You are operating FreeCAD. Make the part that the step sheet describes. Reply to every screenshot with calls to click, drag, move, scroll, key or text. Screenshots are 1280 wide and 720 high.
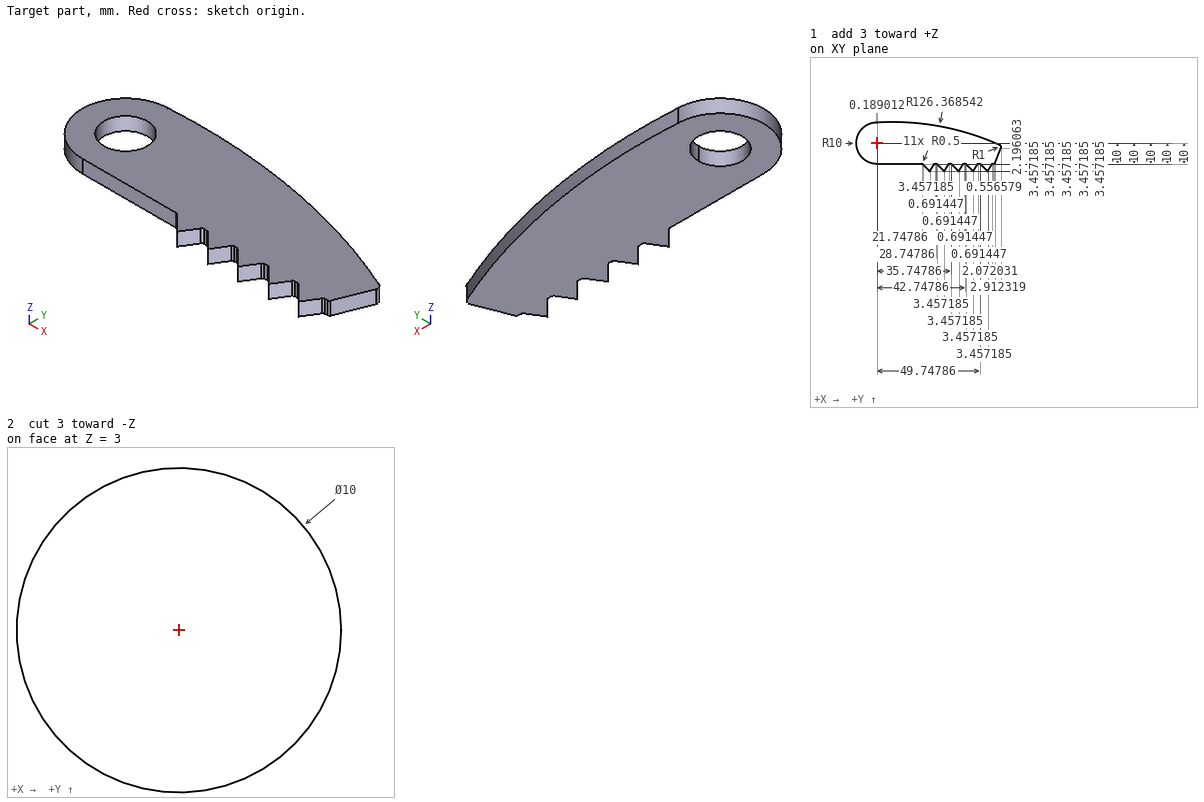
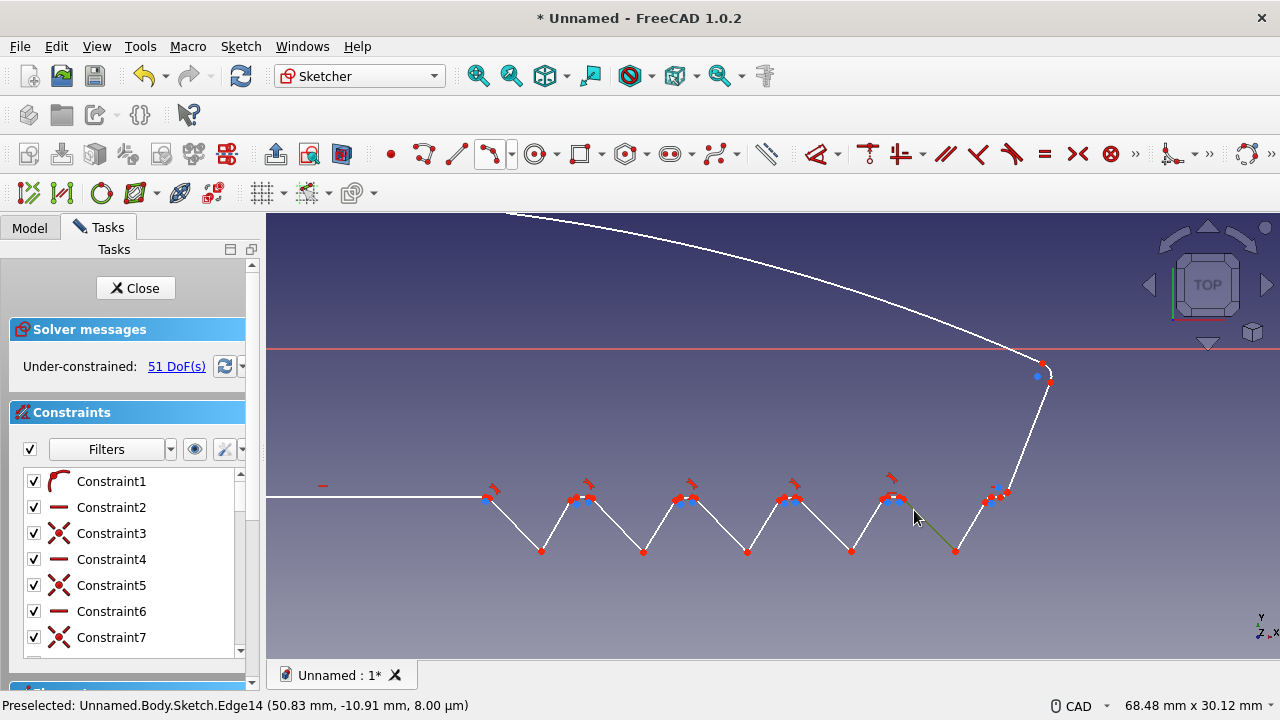
scroll(902, 498, up, 9)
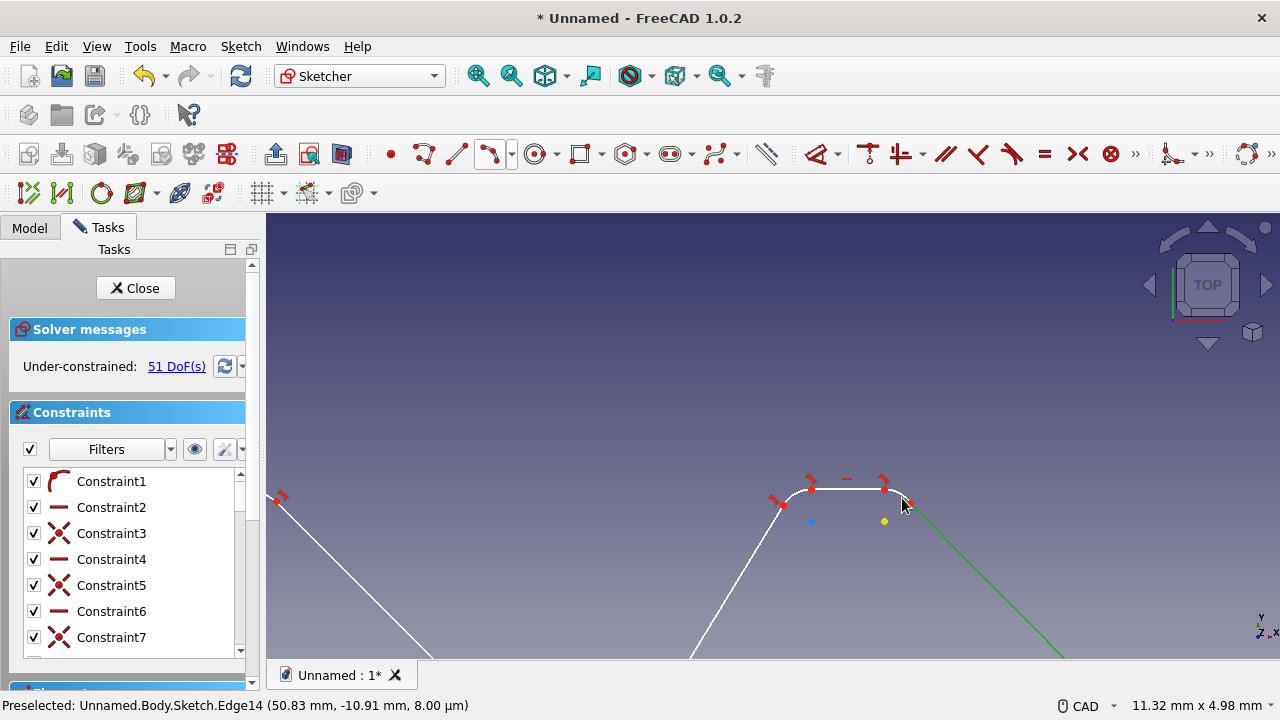
click(899, 493)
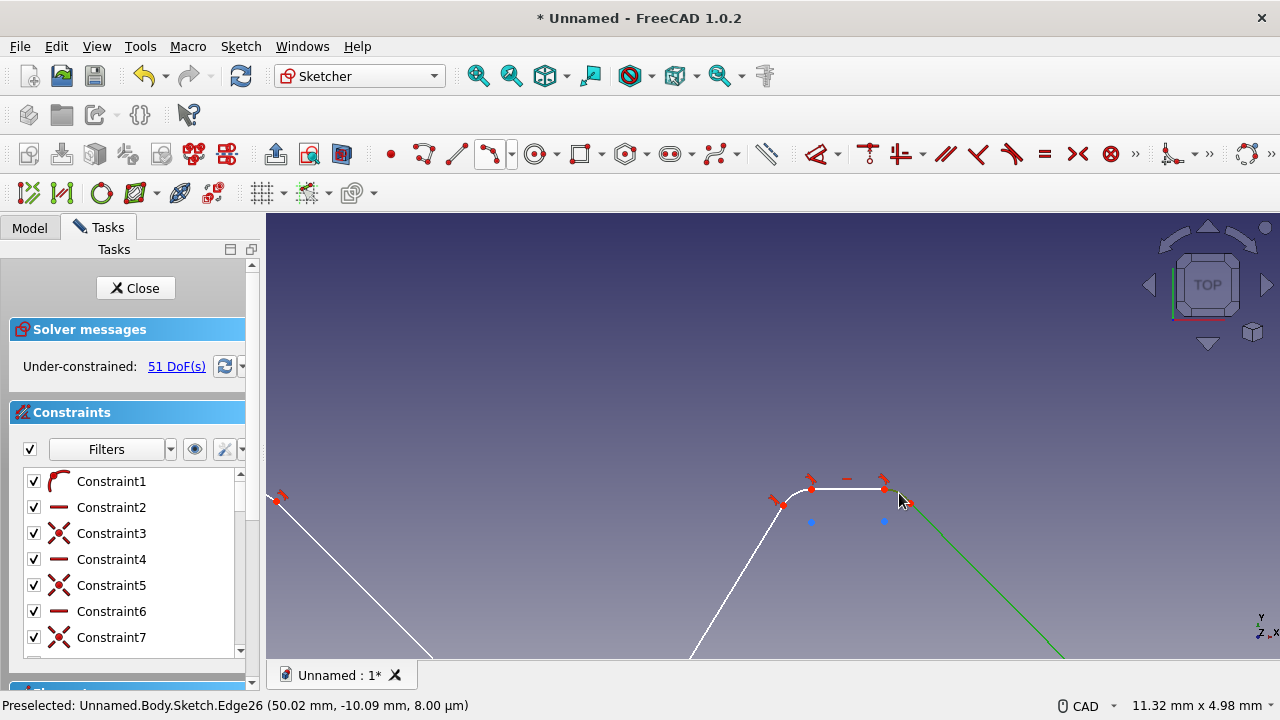
click(1012, 154)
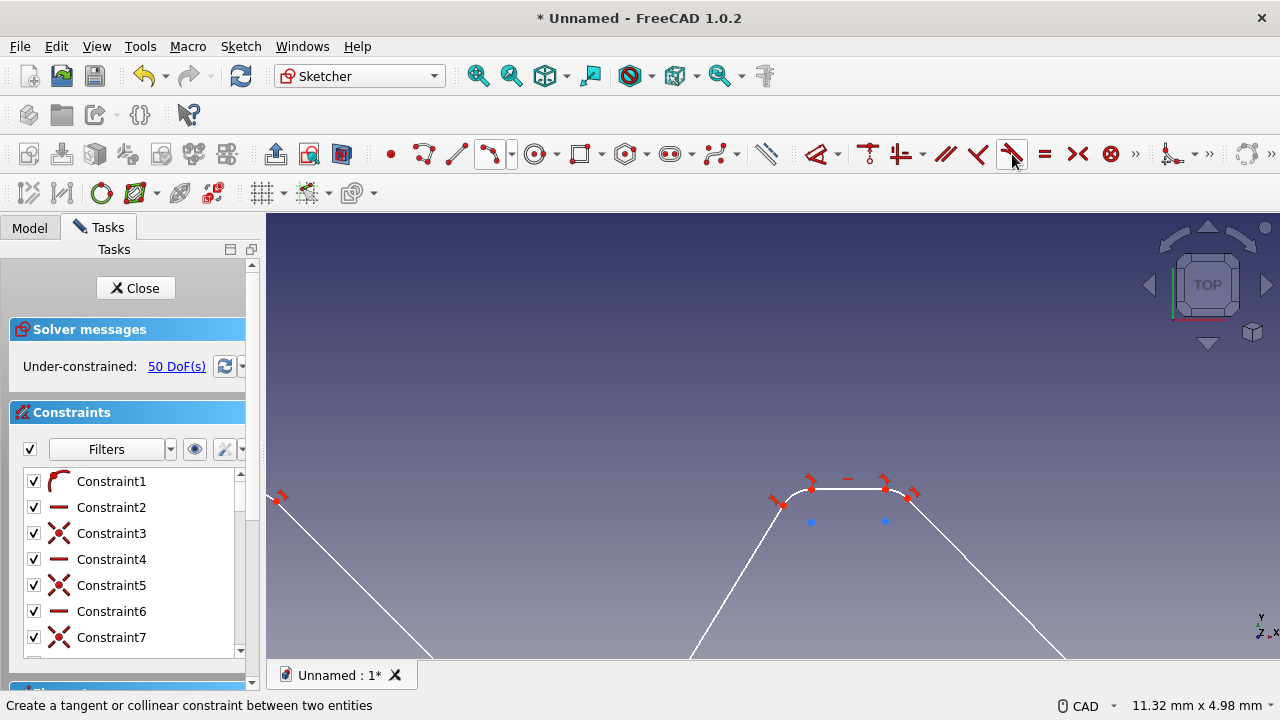
scroll(908, 504, down, 12)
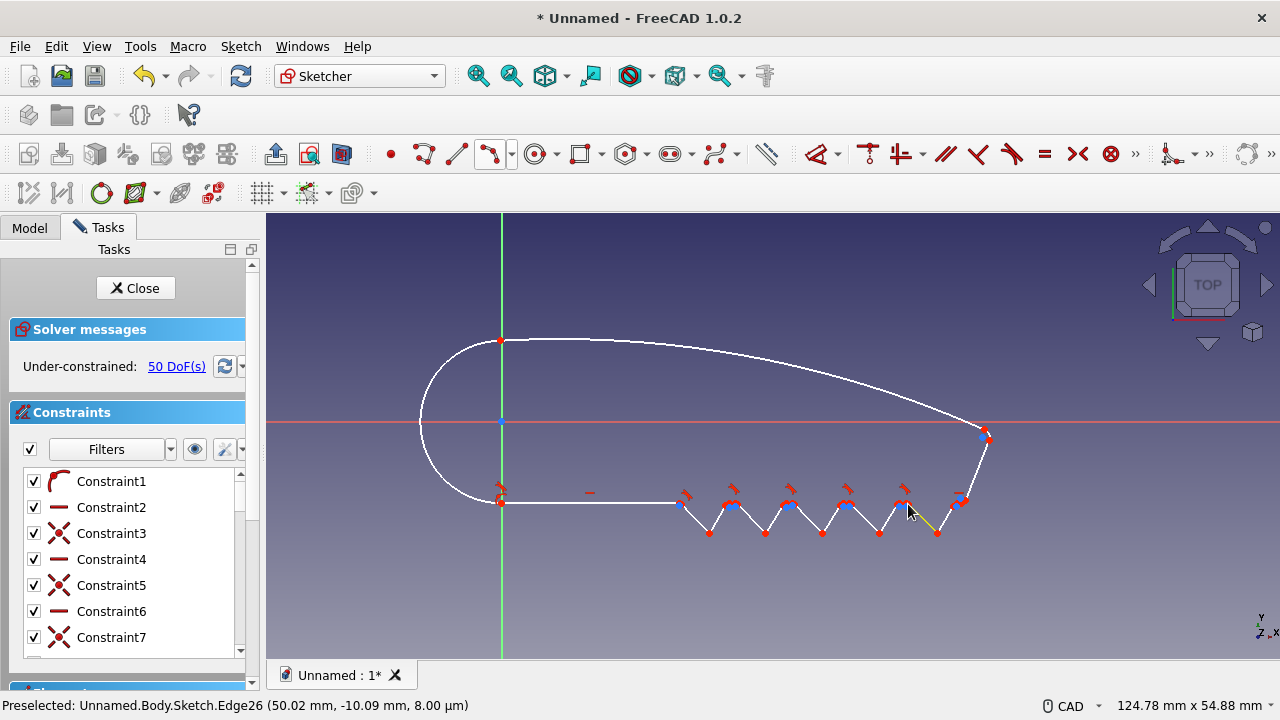
scroll(942, 525, up, 3)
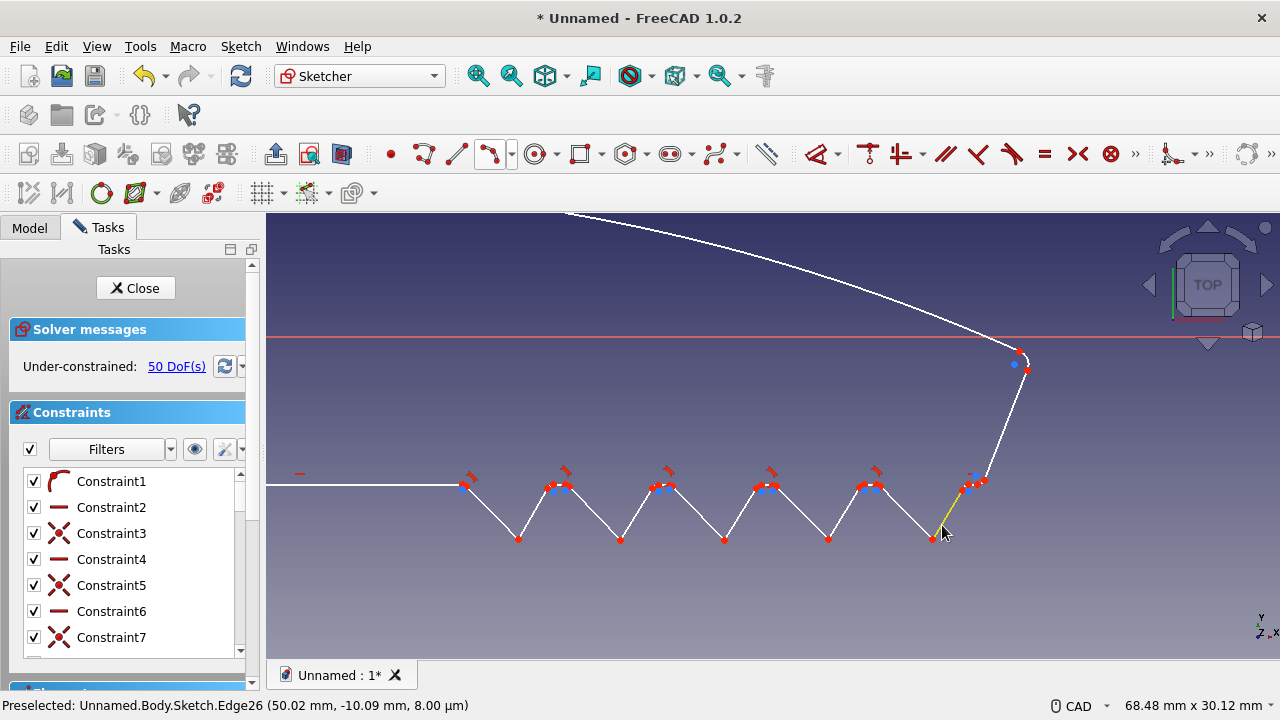
click(942, 525)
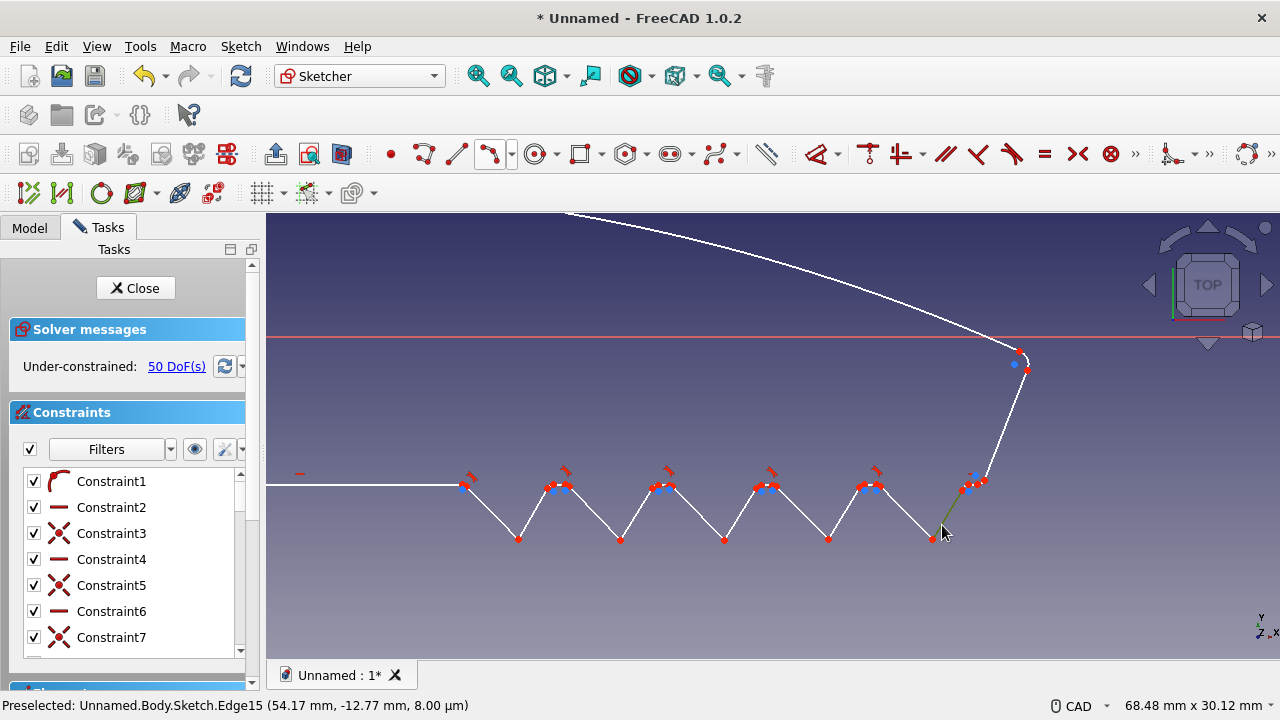
scroll(964, 486, up, 6)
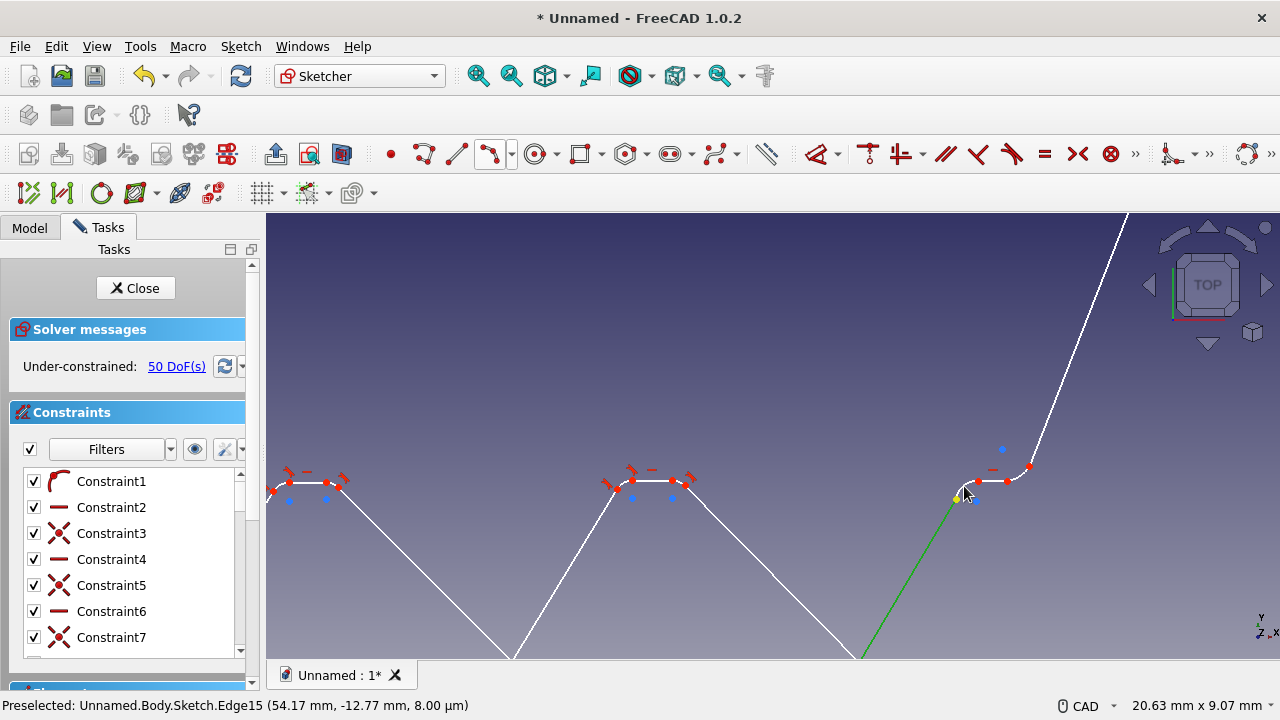
click(964, 485)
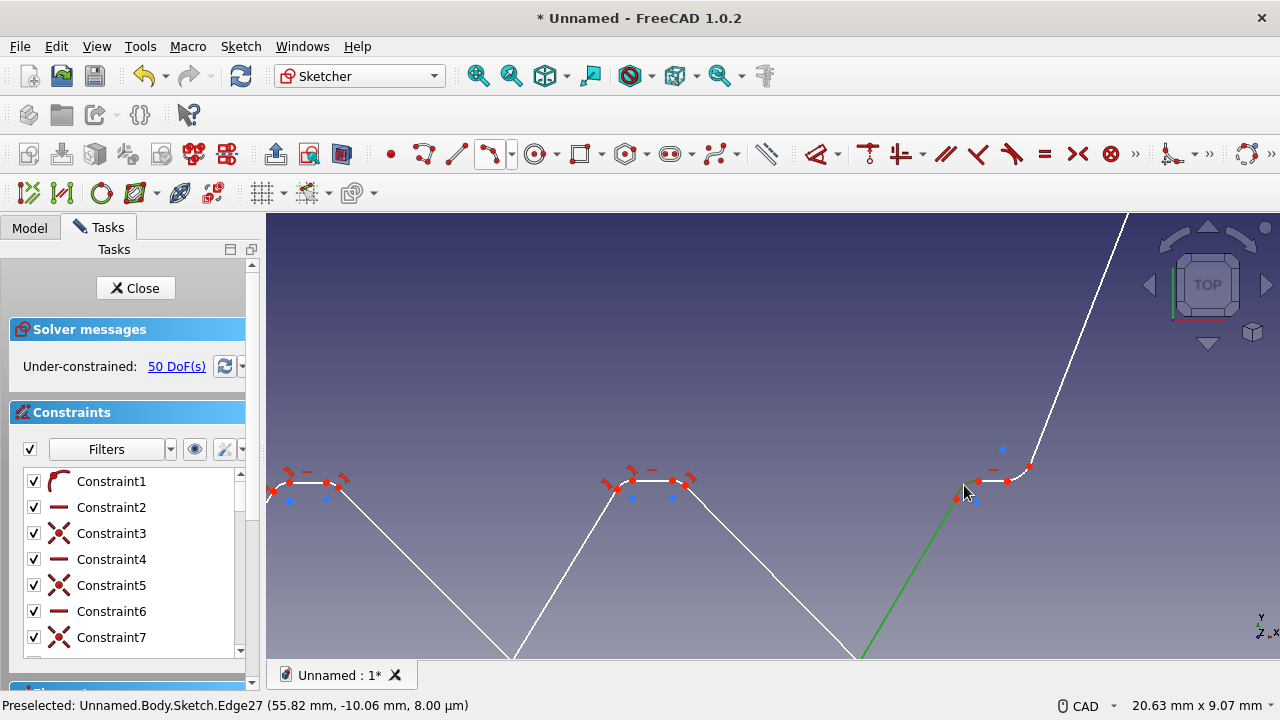
key(t)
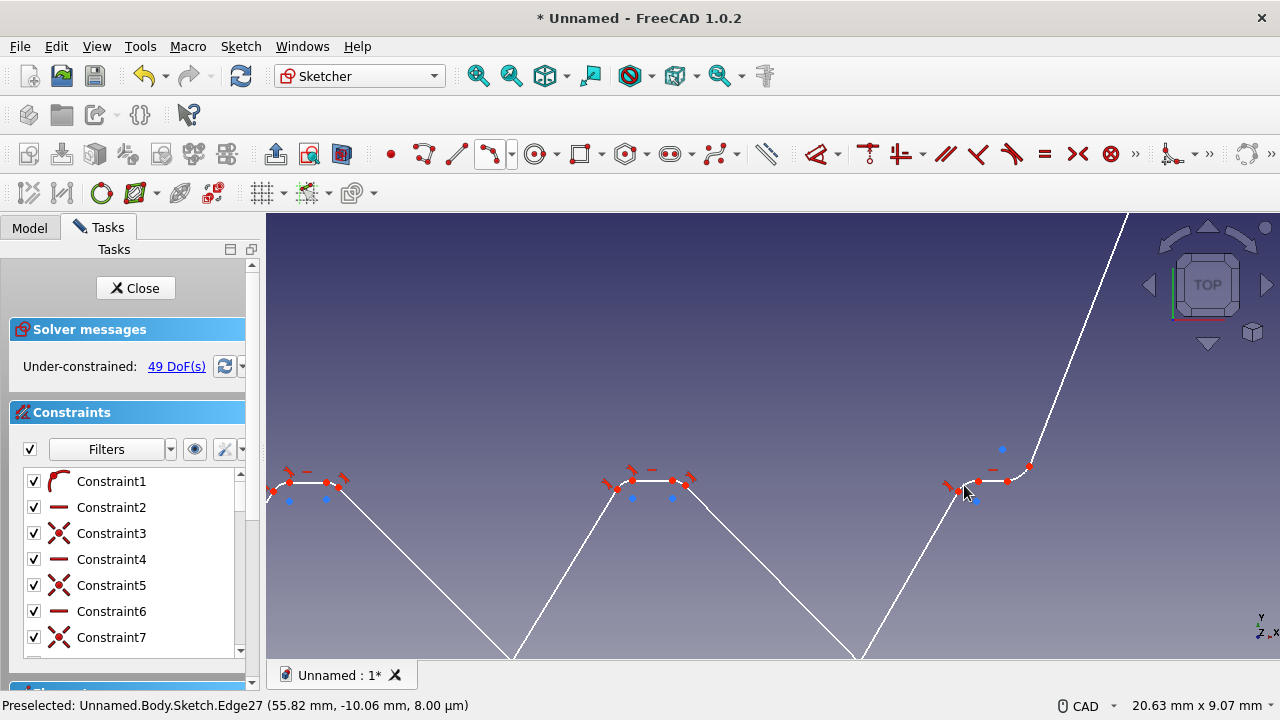
click(990, 481)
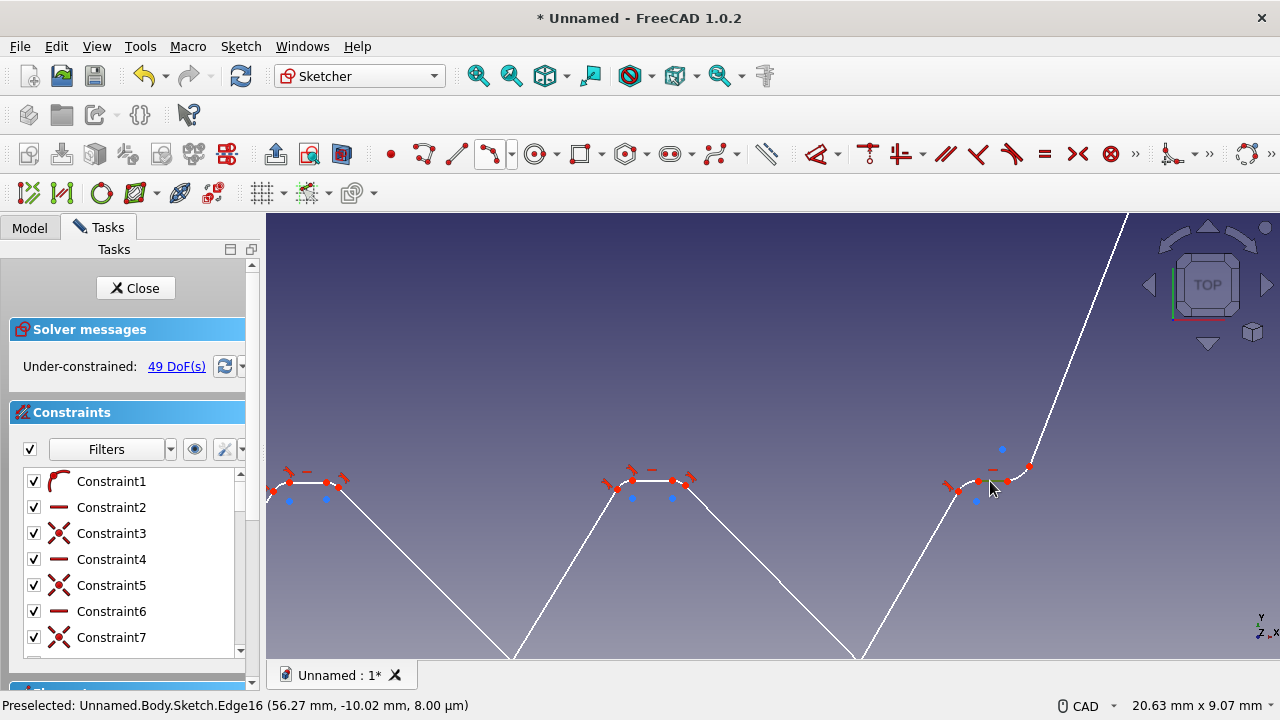
click(967, 483)